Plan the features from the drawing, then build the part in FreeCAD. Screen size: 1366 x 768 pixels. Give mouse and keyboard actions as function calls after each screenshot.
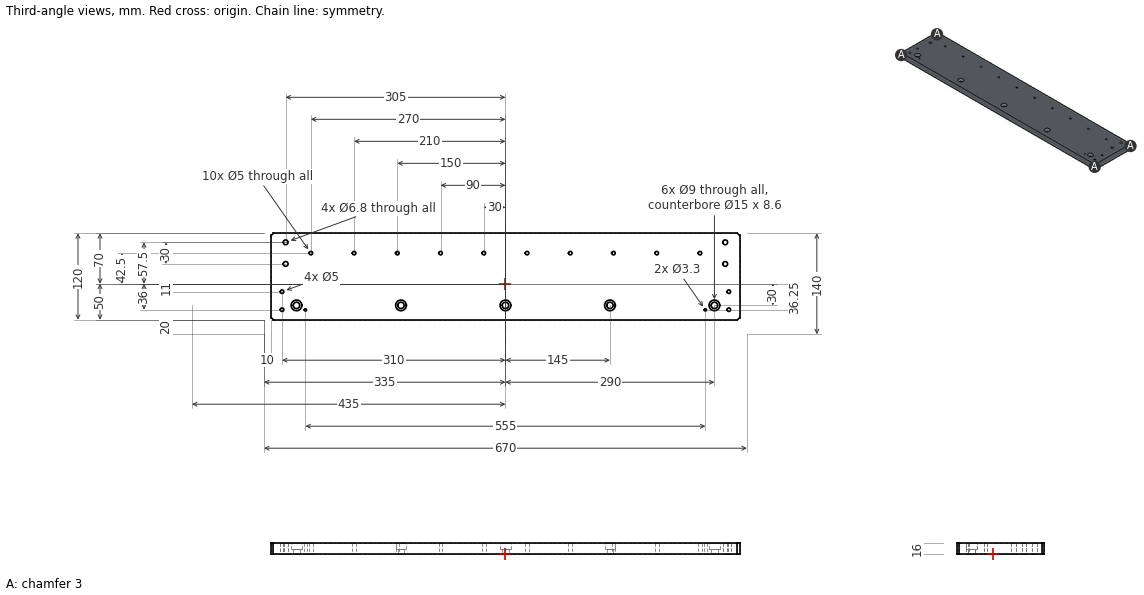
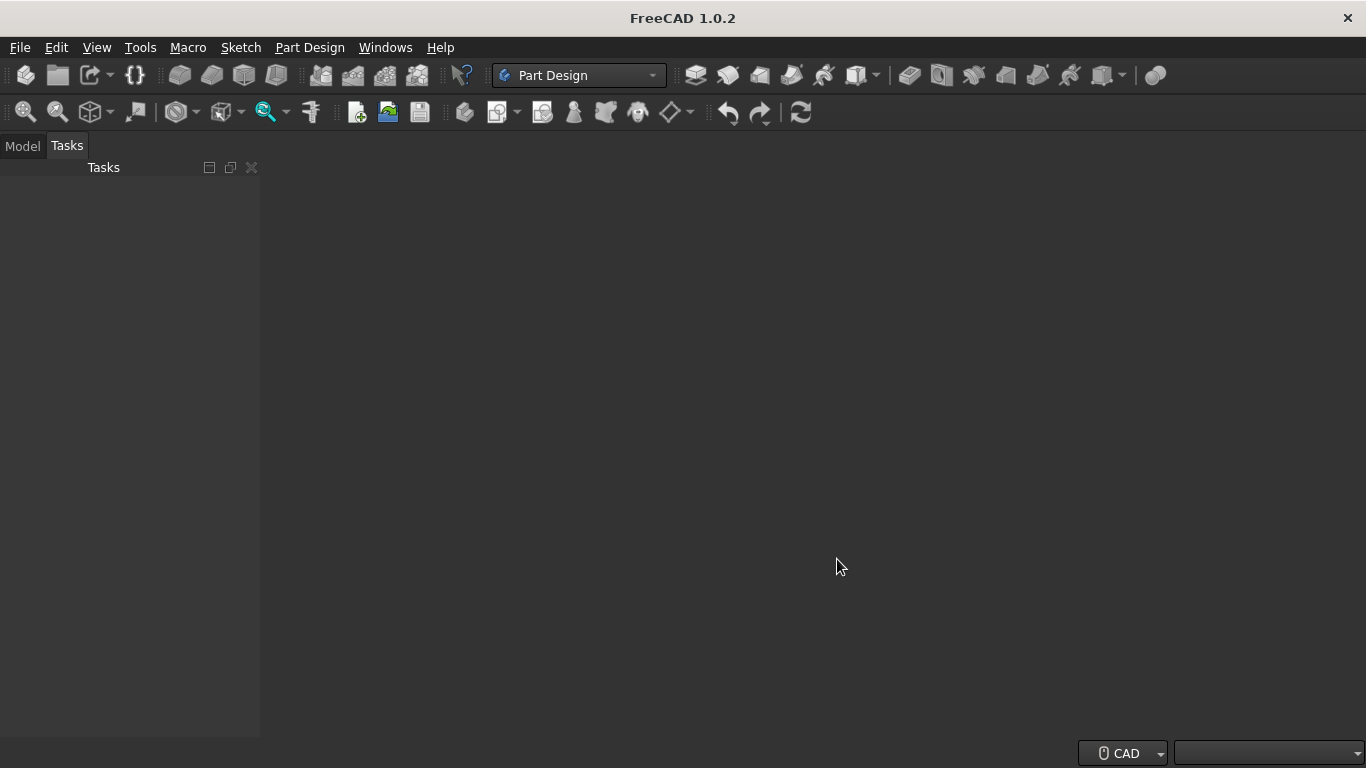
click(356, 112)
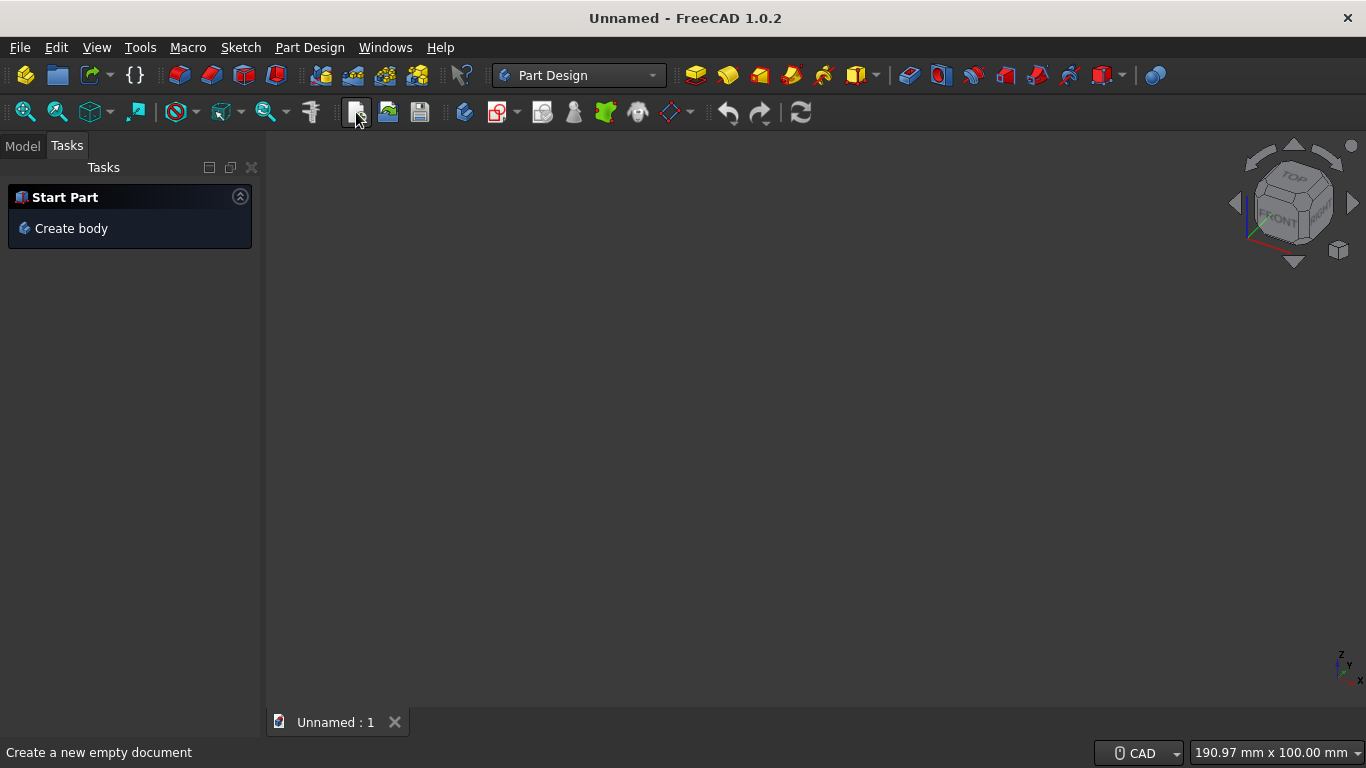
click(498, 112)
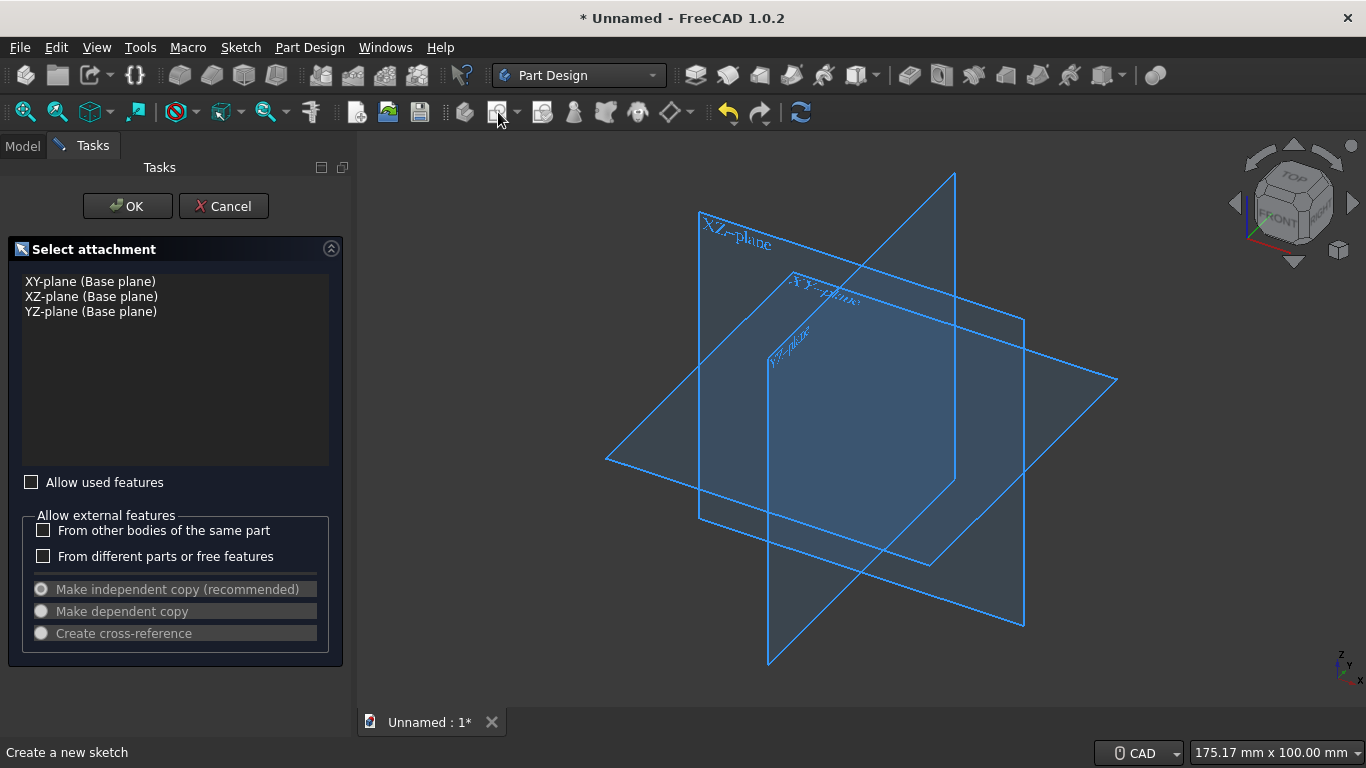
click(82, 282)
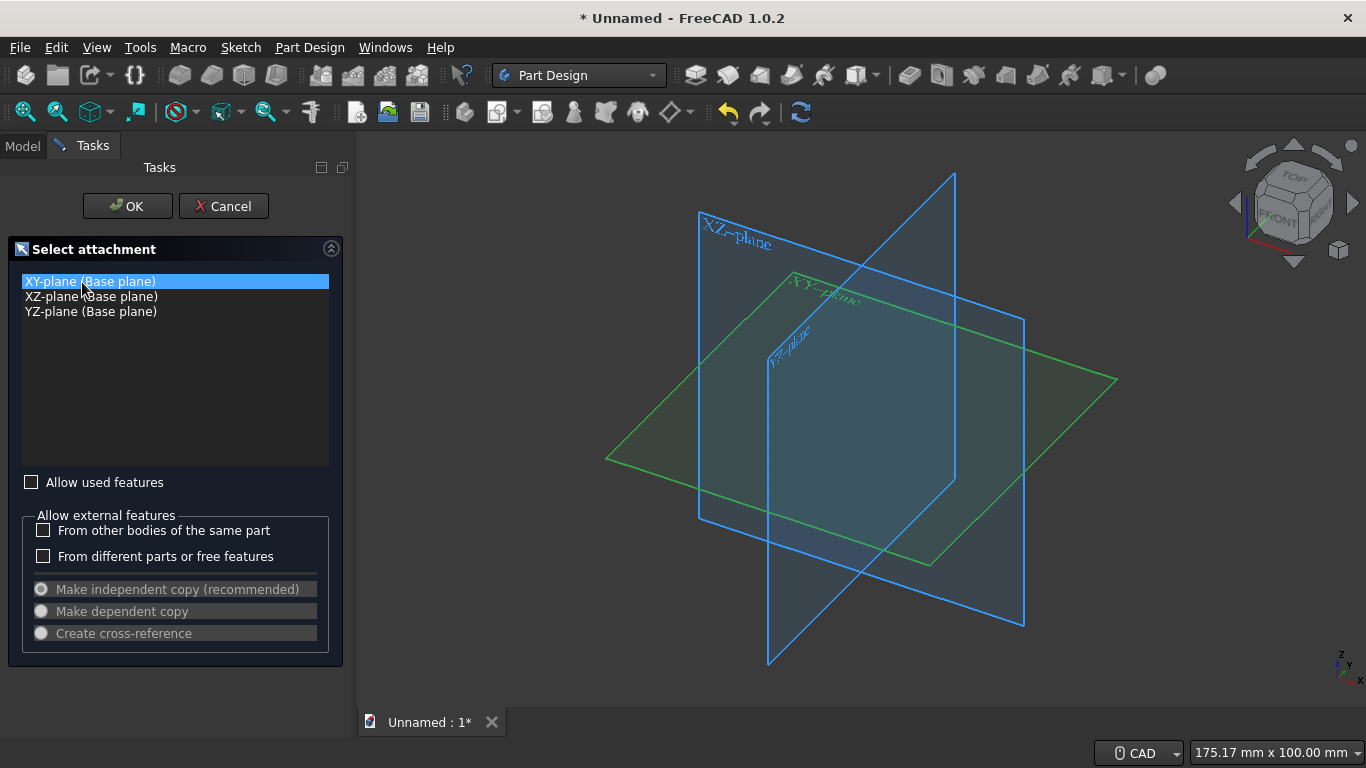
click(128, 206)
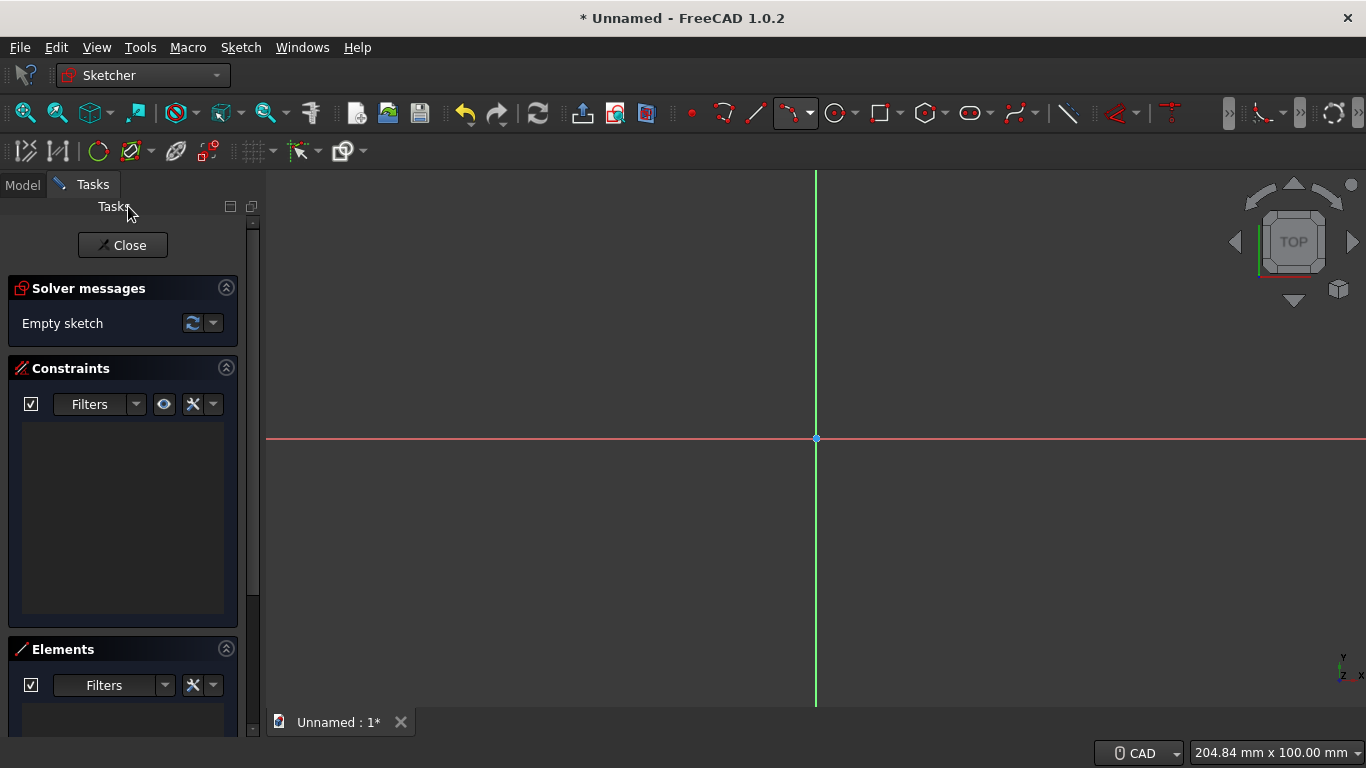
scroll(734, 438, down, 9)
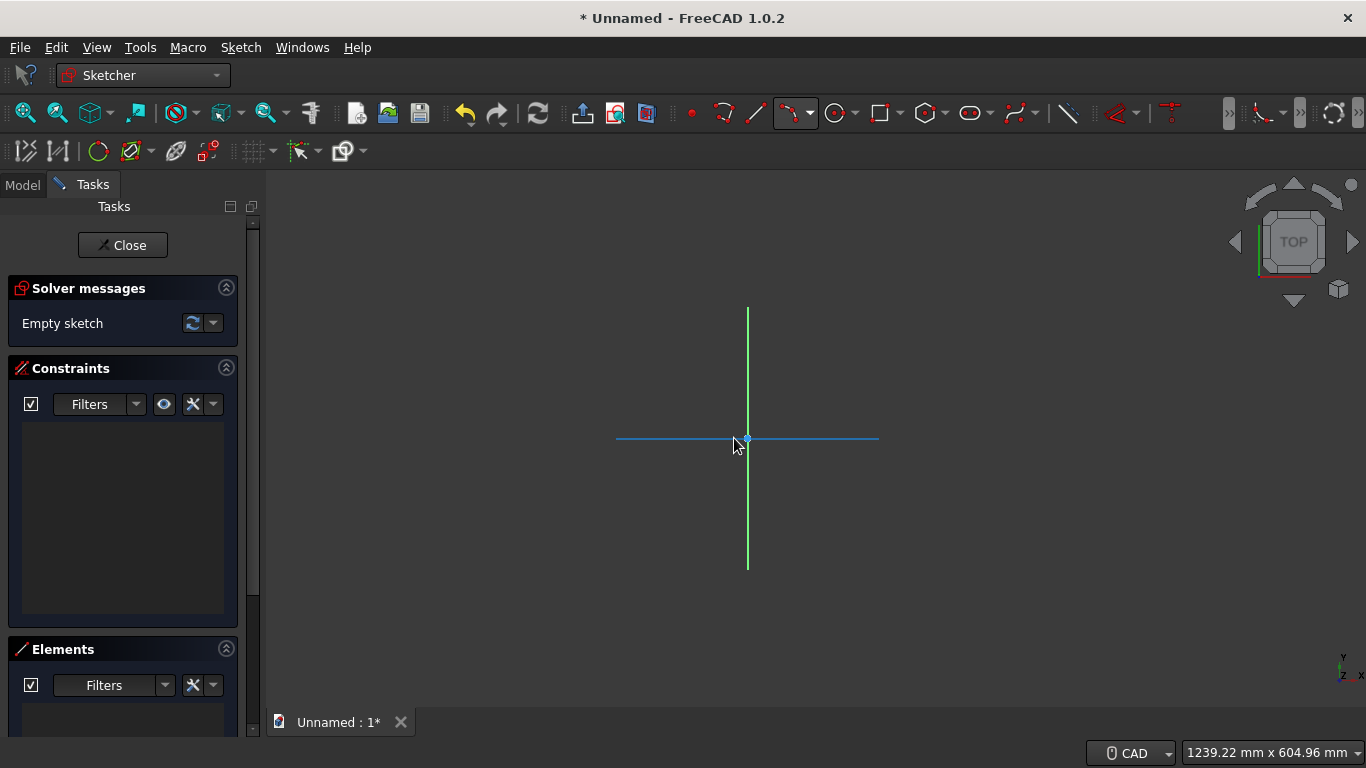
click(902, 114)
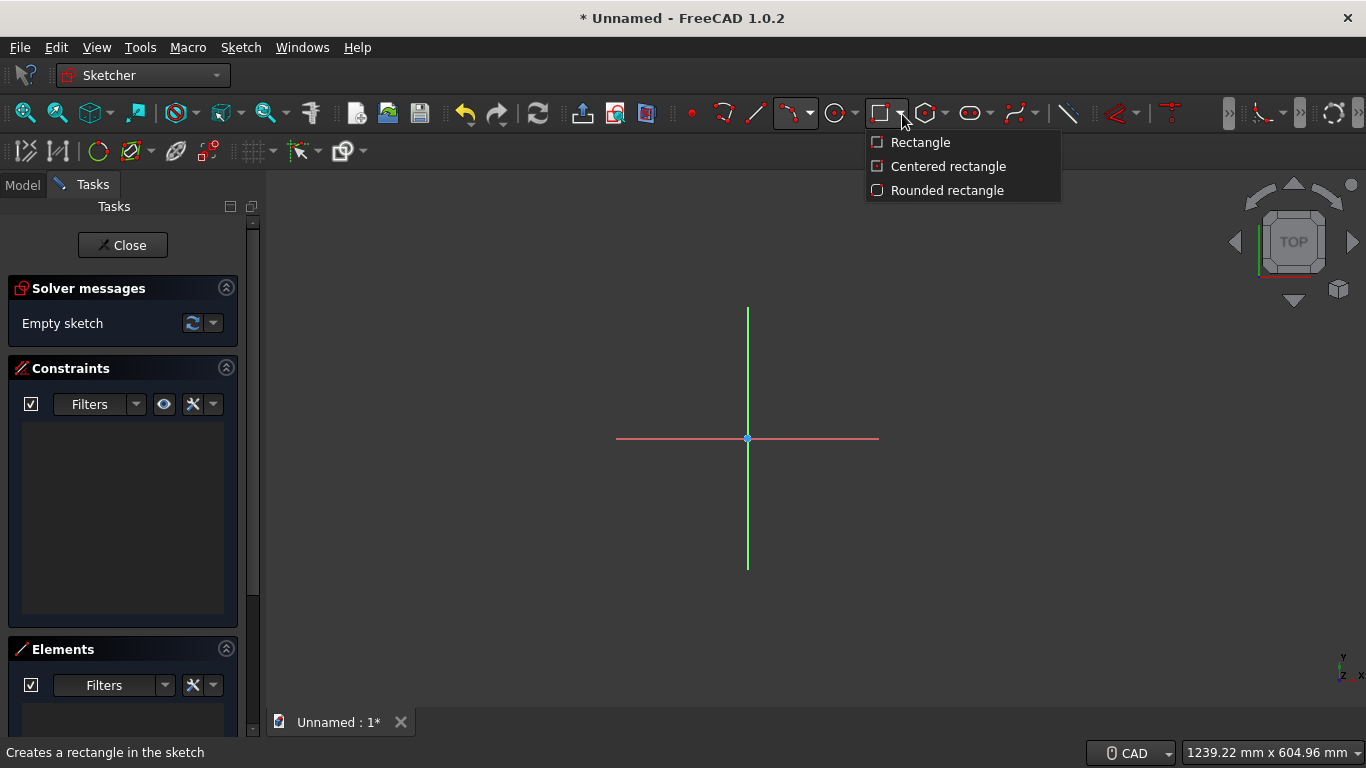
click(964, 166)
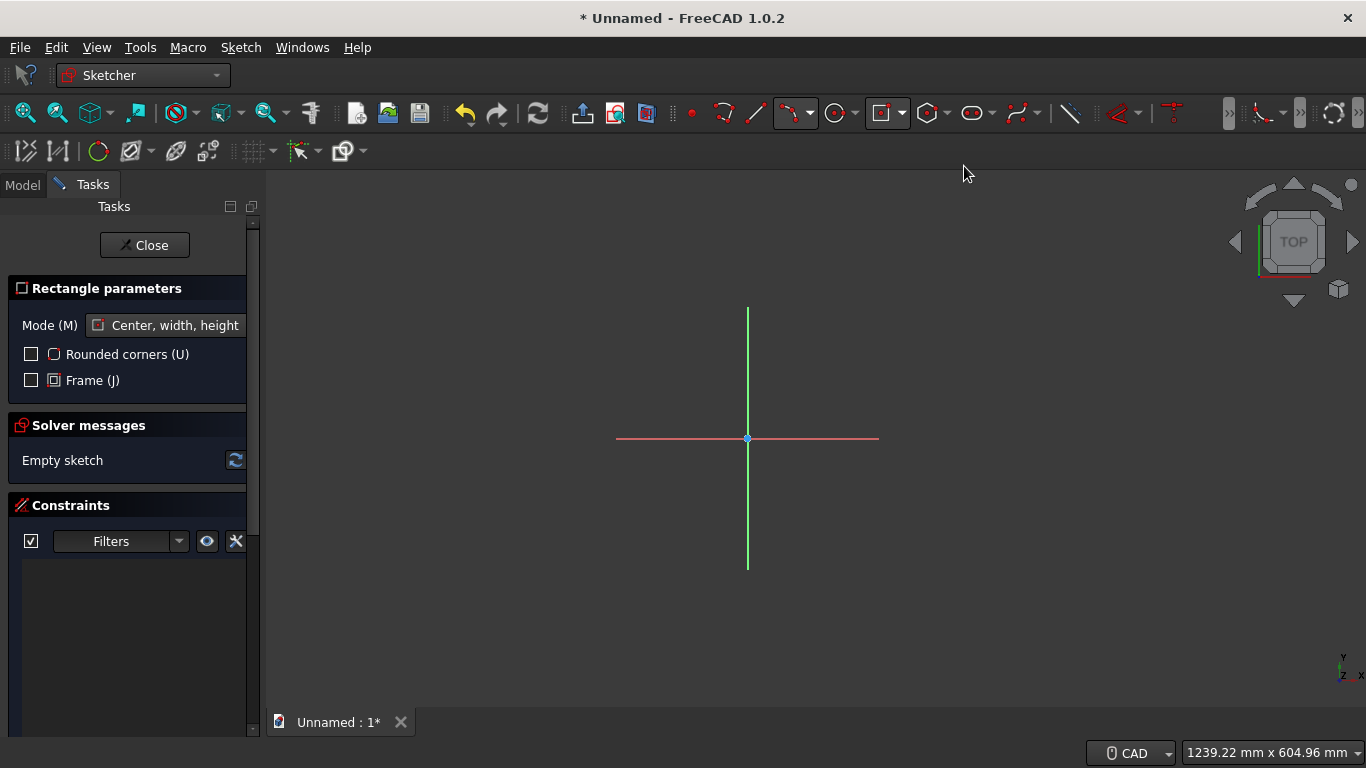
click(748, 438)
click(1045, 376)
key(Escape)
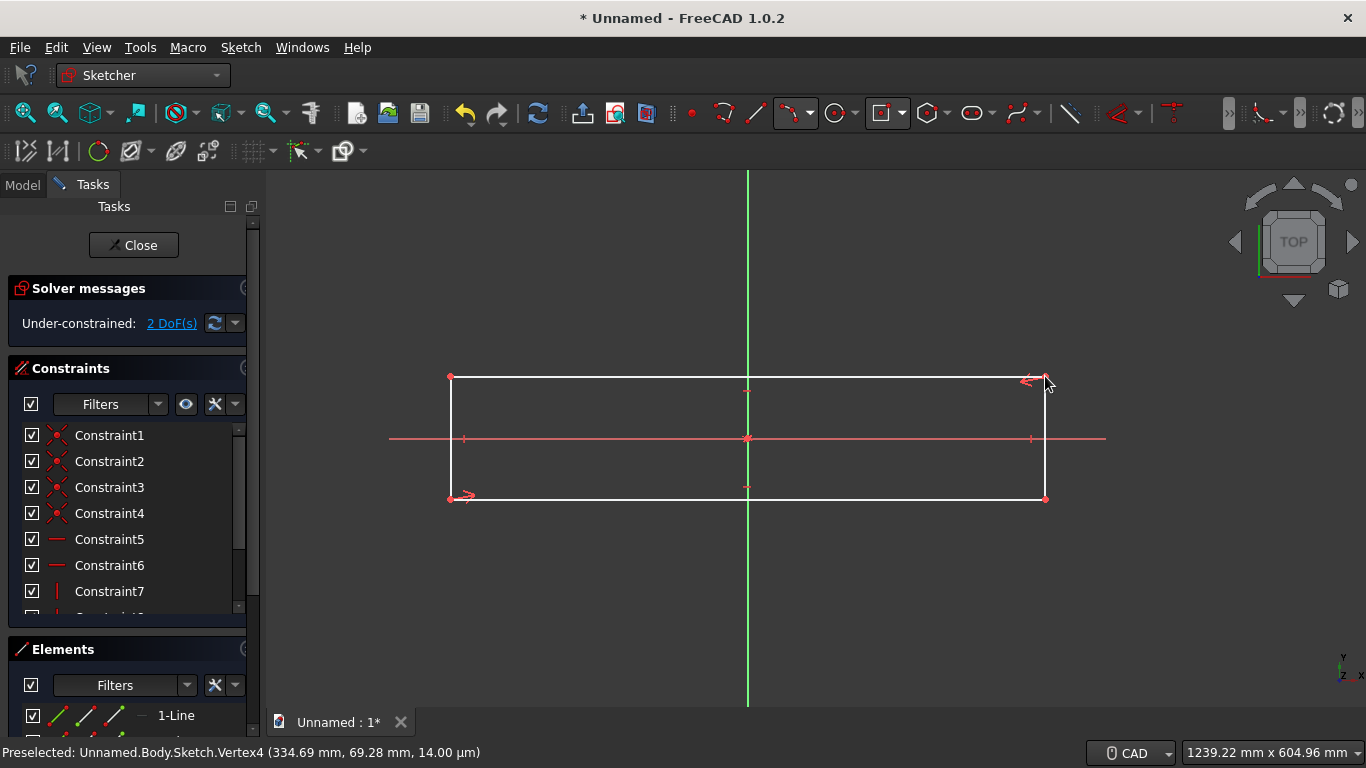
click(629, 500)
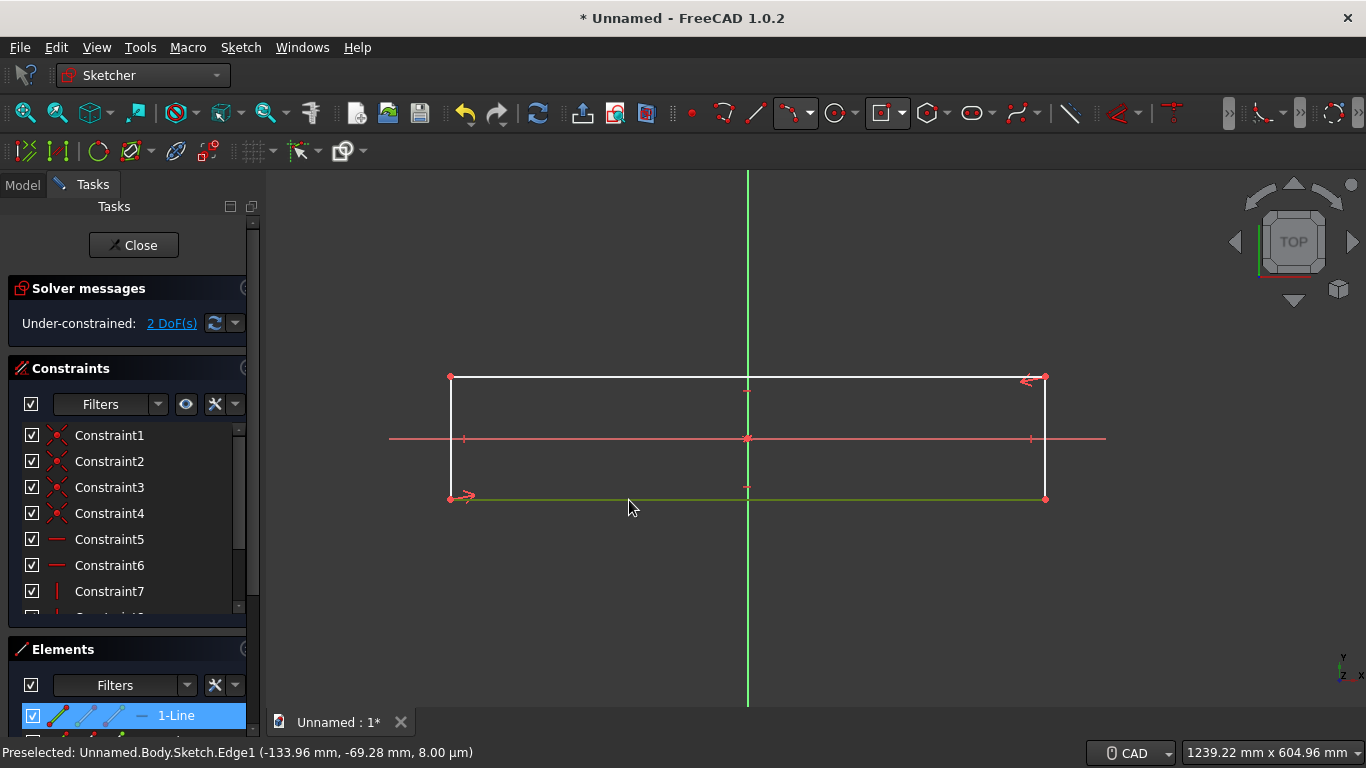
click(1140, 114)